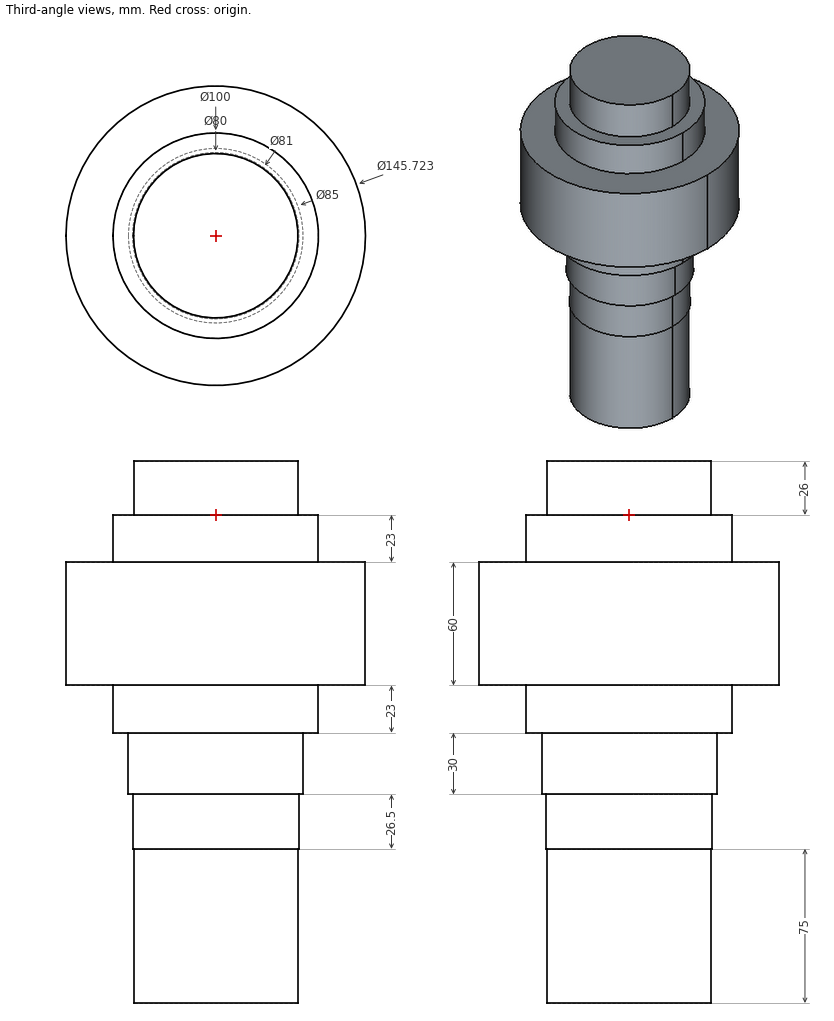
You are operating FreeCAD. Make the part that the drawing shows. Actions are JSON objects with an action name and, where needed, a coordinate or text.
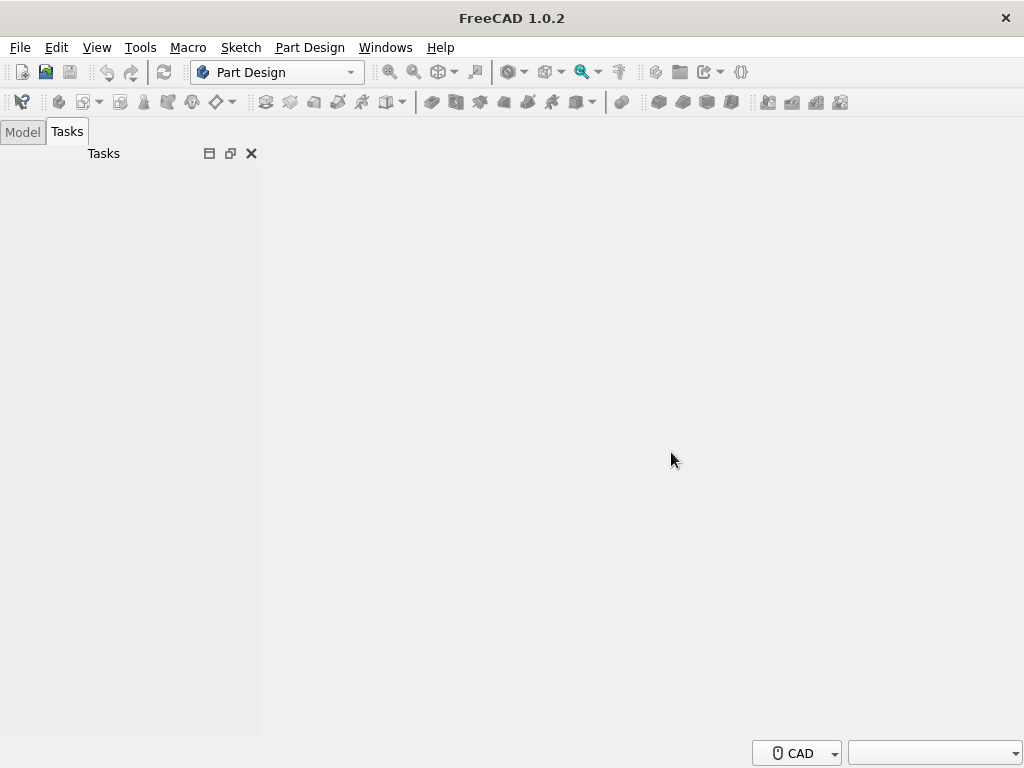
{"action": "key", "text": "ctrl+n"}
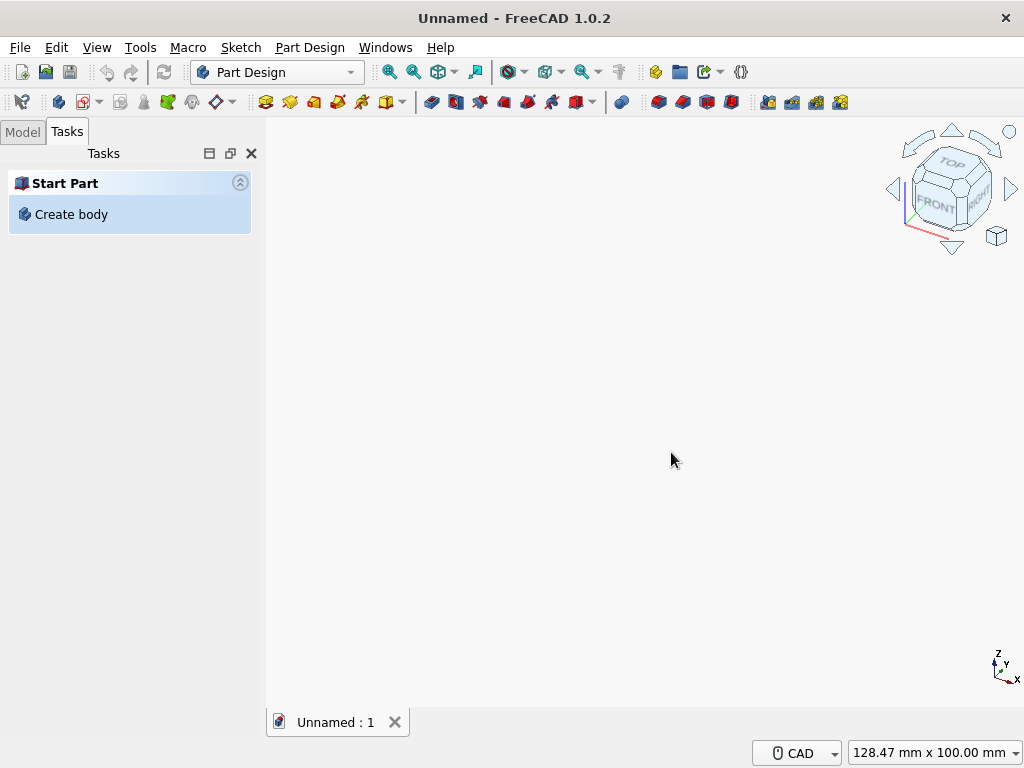
{"action": "left_click", "coordinate": [84, 102]}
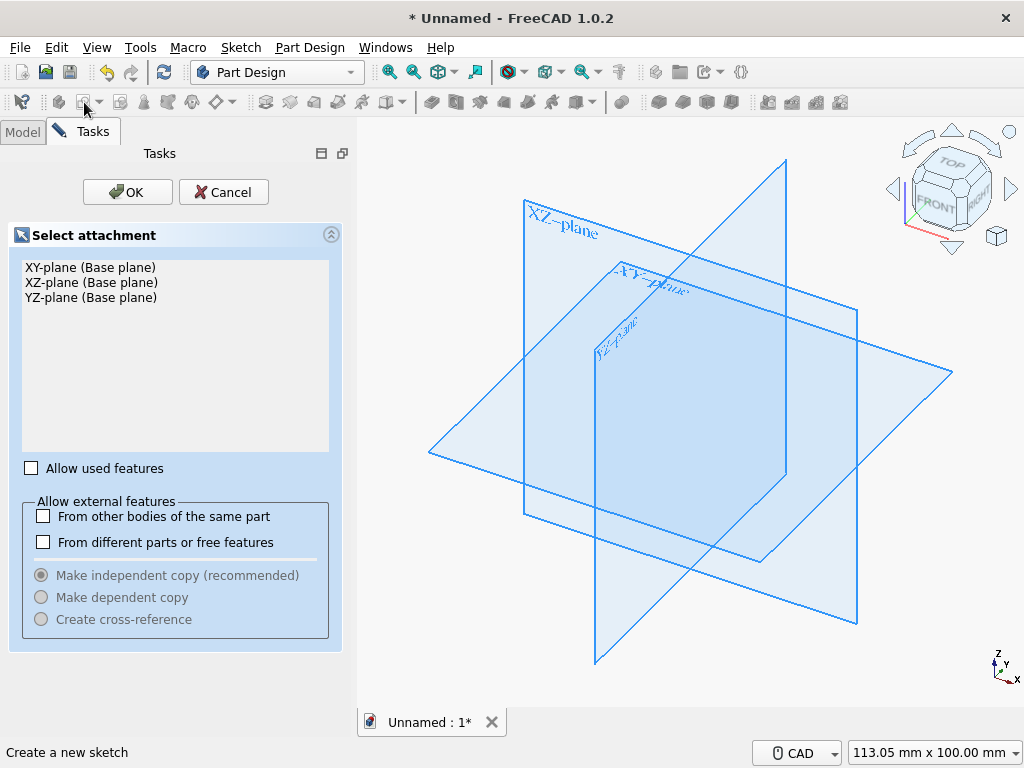
{"action": "left_click", "coordinate": [82, 268]}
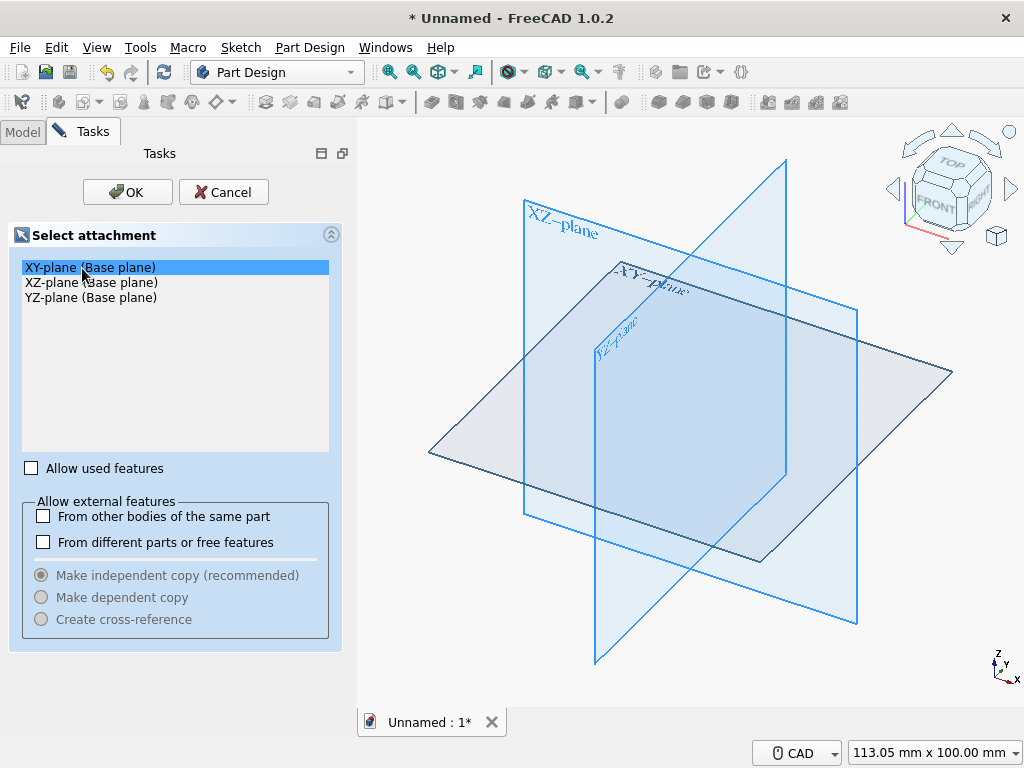
{"action": "left_click", "coordinate": [128, 192]}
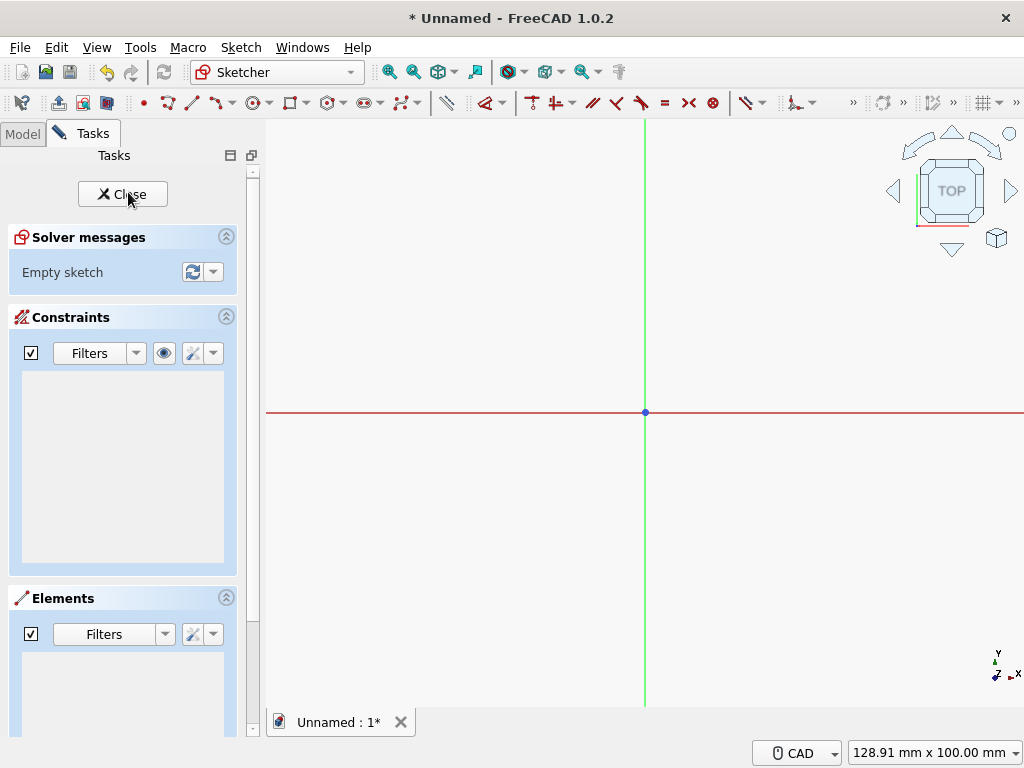
{"action": "scroll", "coordinate": [294, 413], "scroll_direction": "down", "scroll_amount": 1}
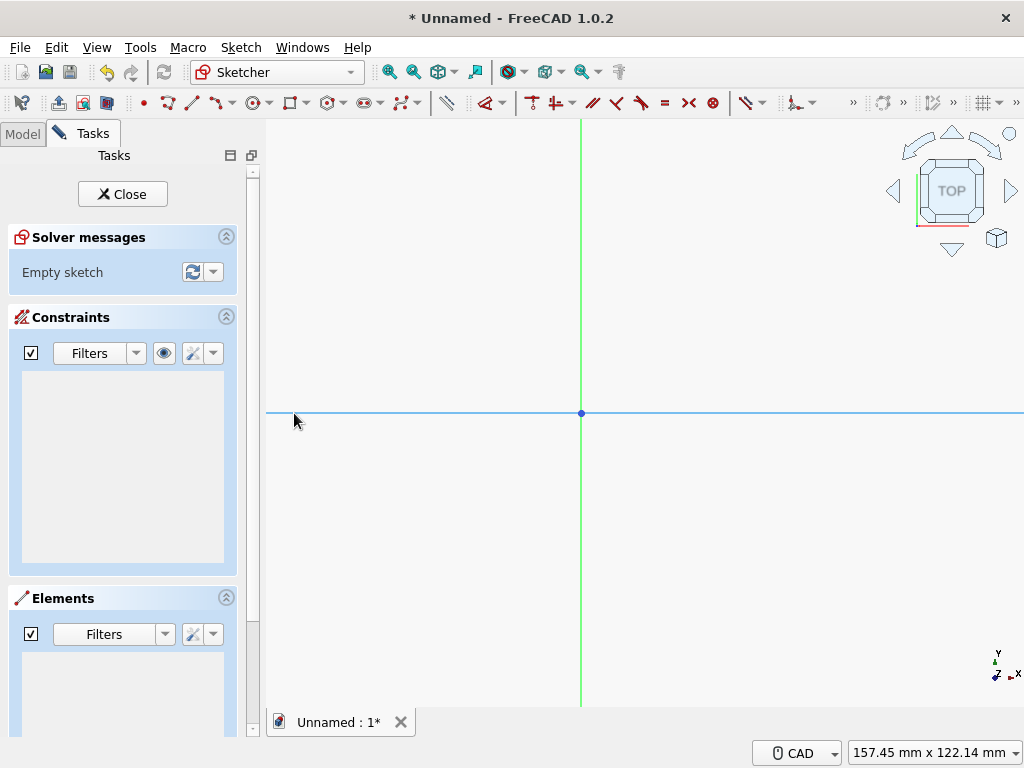
{"action": "left_click", "coordinate": [254, 104]}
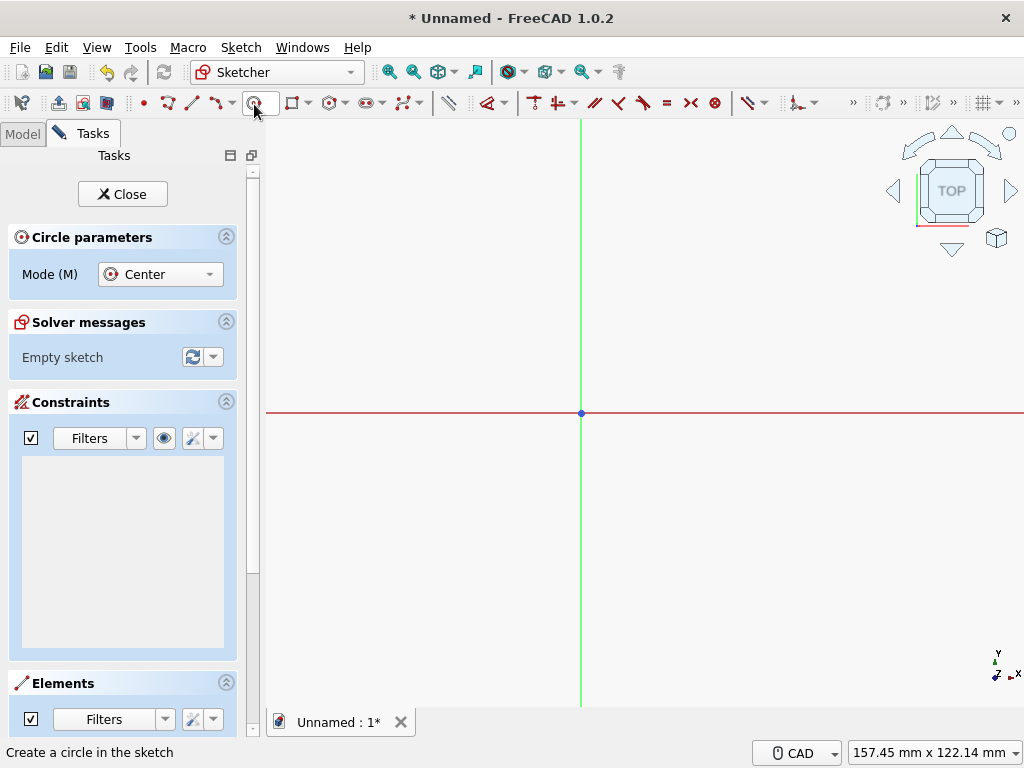
{"action": "left_click", "coordinate": [581, 413]}
{"action": "left_click", "coordinate": [718, 277]}
{"action": "key", "text": "Escape"}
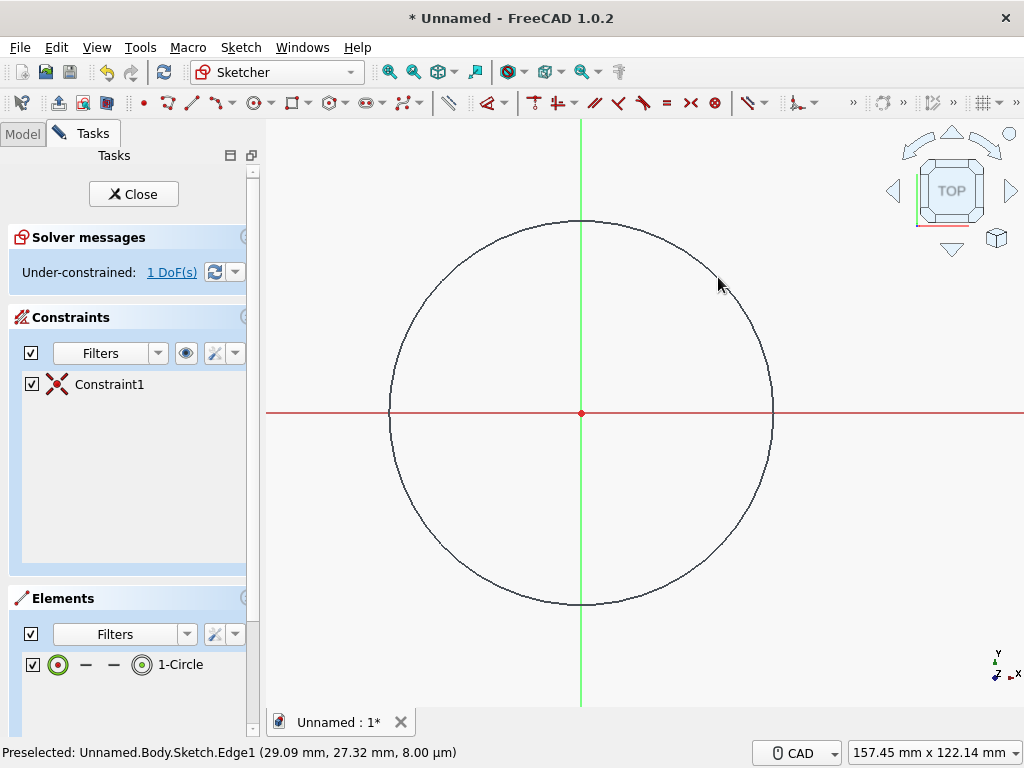
{"action": "key", "text": "d"}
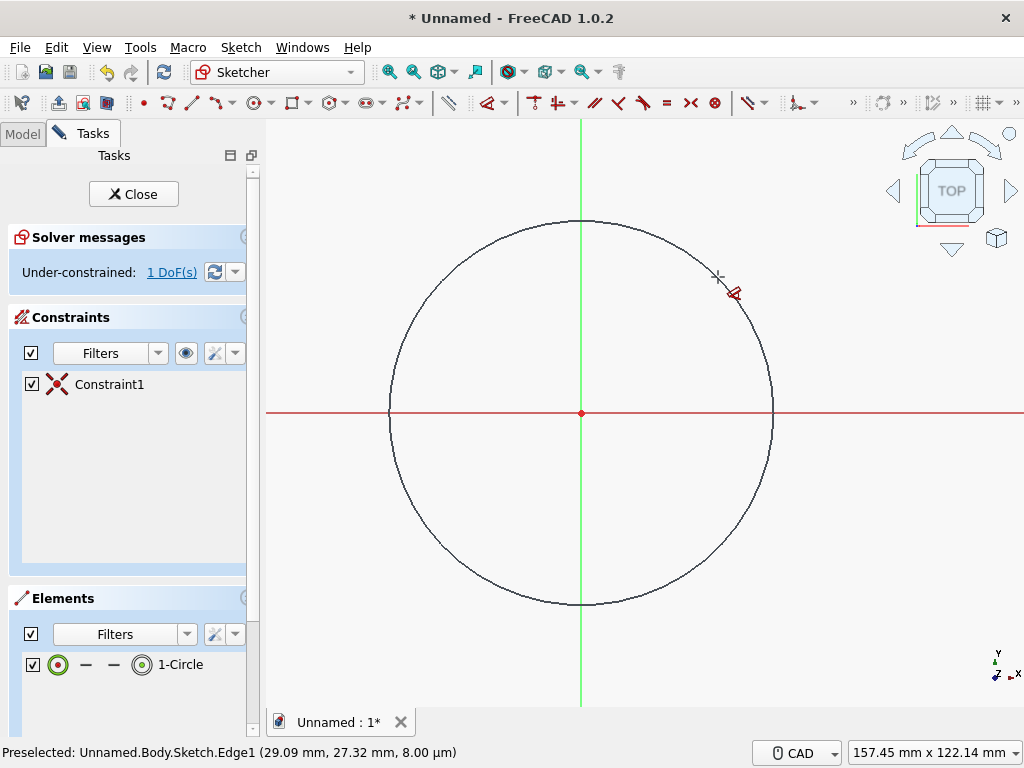
{"action": "left_click", "coordinate": [717, 277]}
{"action": "left_click", "coordinate": [740, 254]}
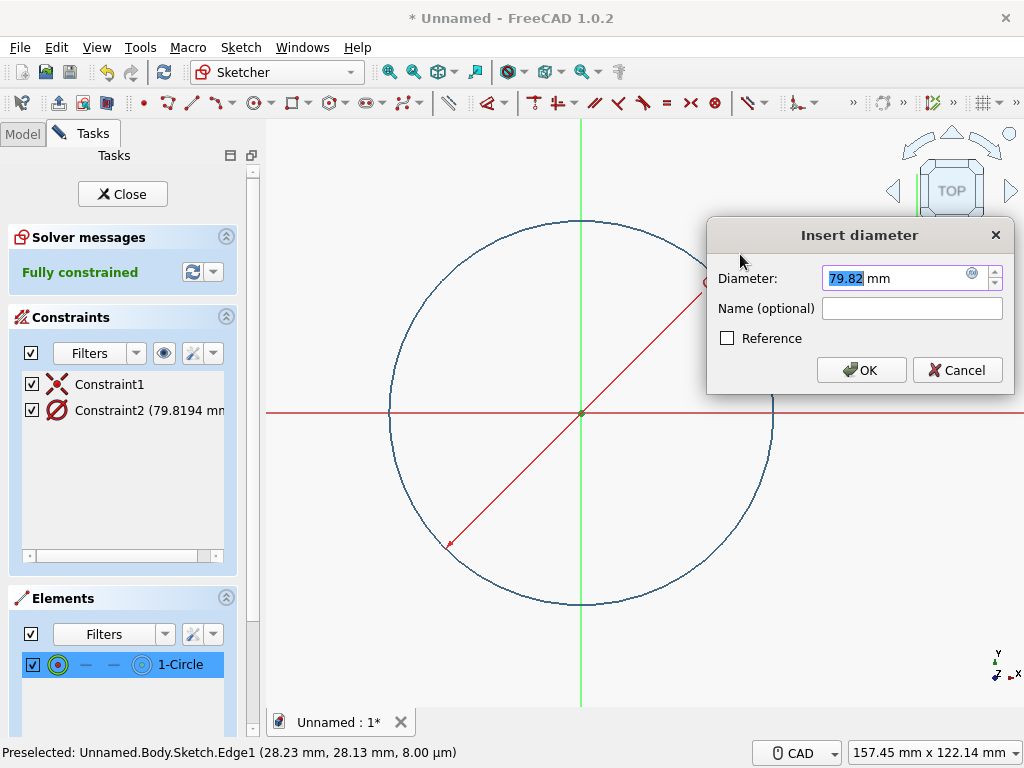
{"action": "type", "text": "80"}
{"action": "key", "text": "Return"}
{"action": "key", "text": "Escape"}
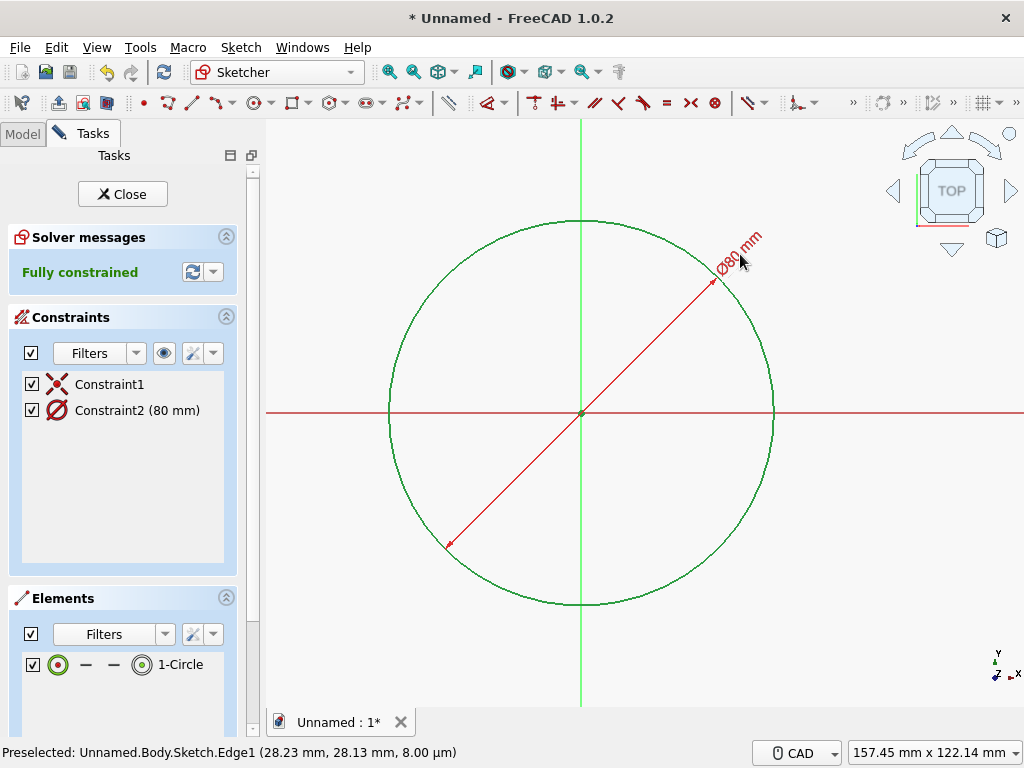
{"action": "left_click", "coordinate": [123, 194]}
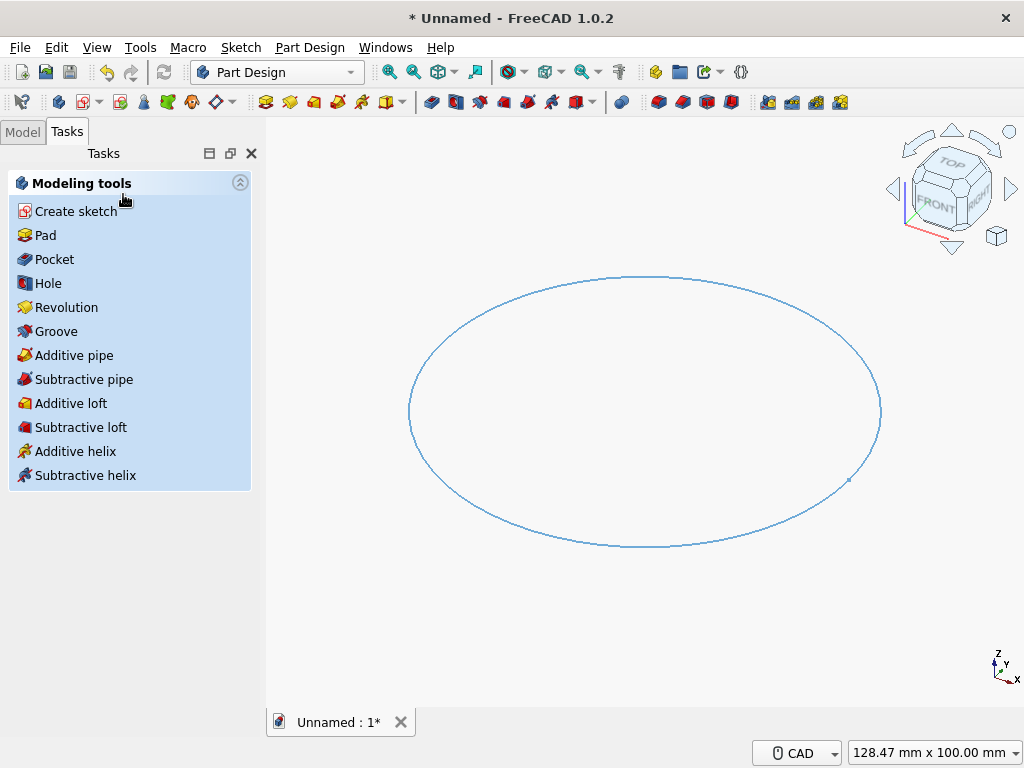
{"action": "left_click", "coordinate": [266, 102]}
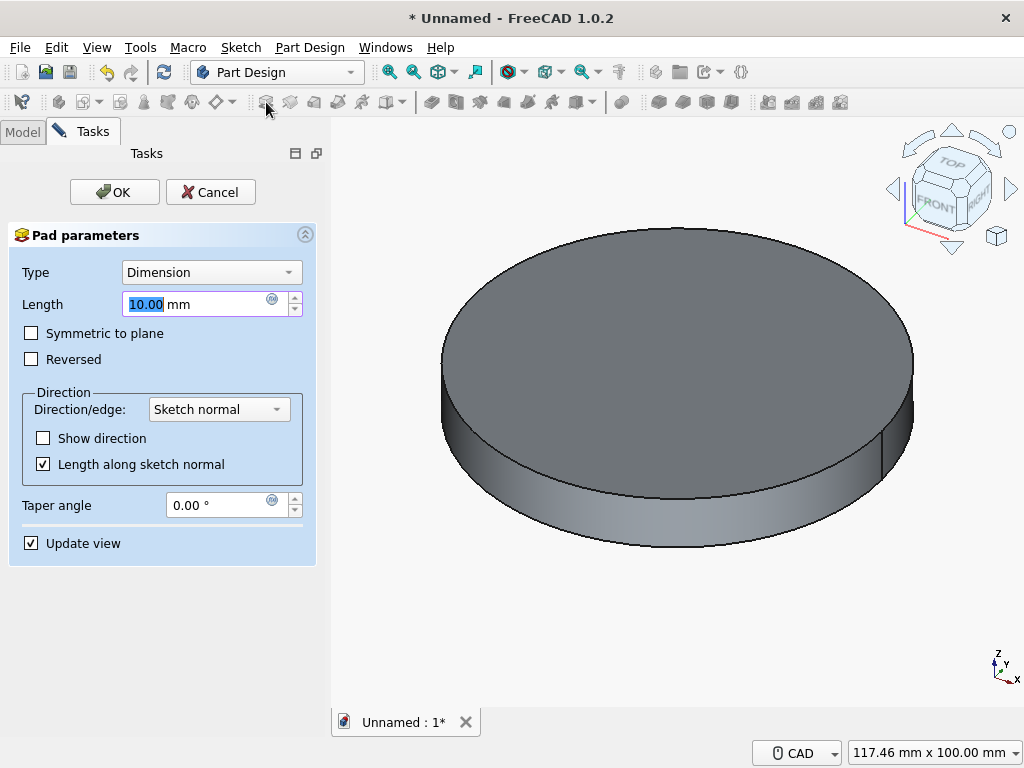
{"action": "type", "text": "26"}
{"action": "key", "text": "Tab"}